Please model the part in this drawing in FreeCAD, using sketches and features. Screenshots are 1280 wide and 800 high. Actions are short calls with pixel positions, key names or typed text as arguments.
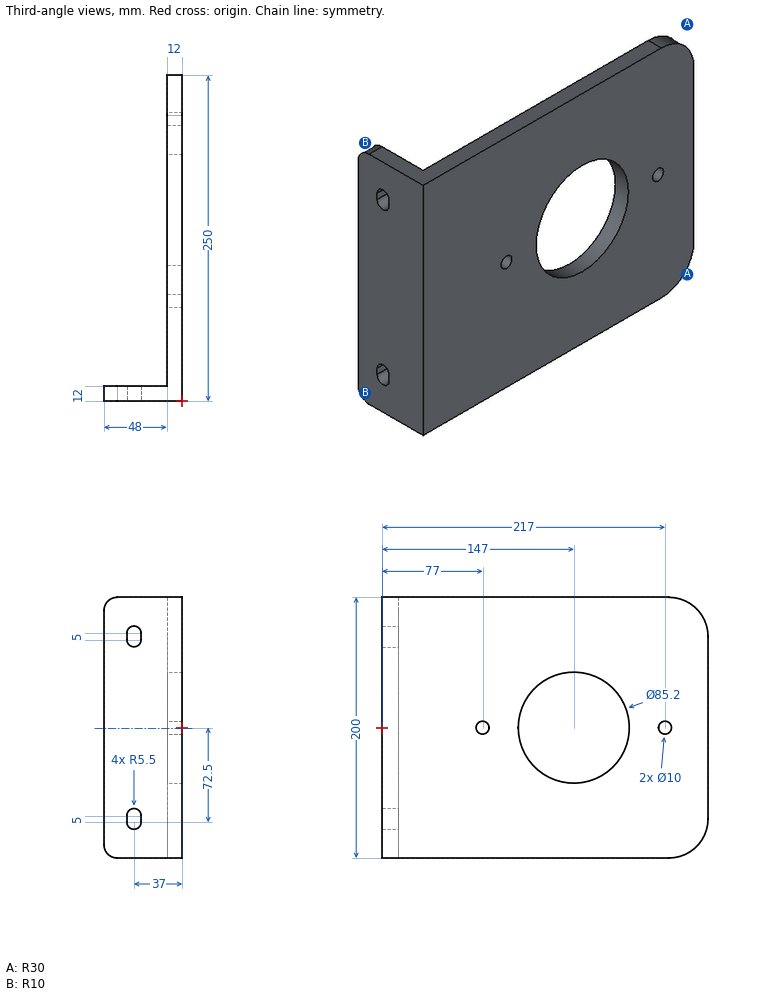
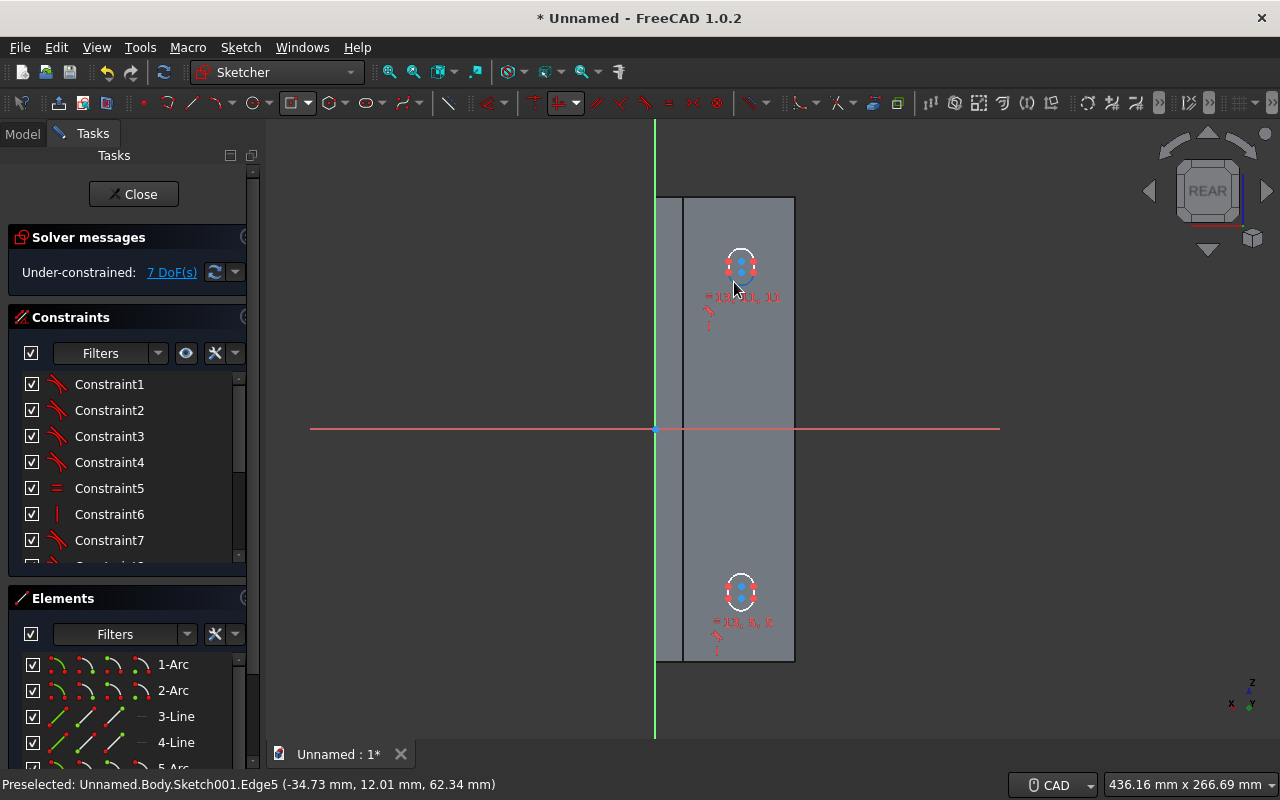
click(741, 587)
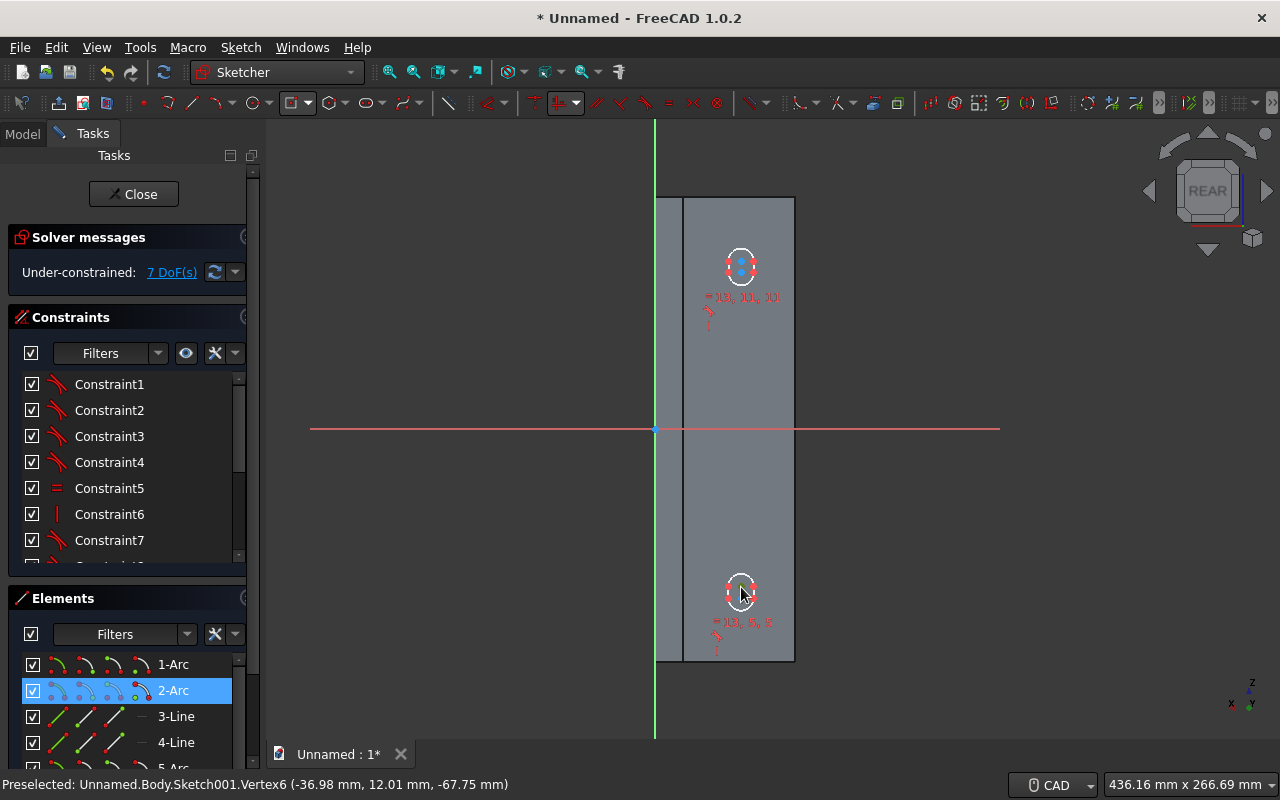
click(741, 273)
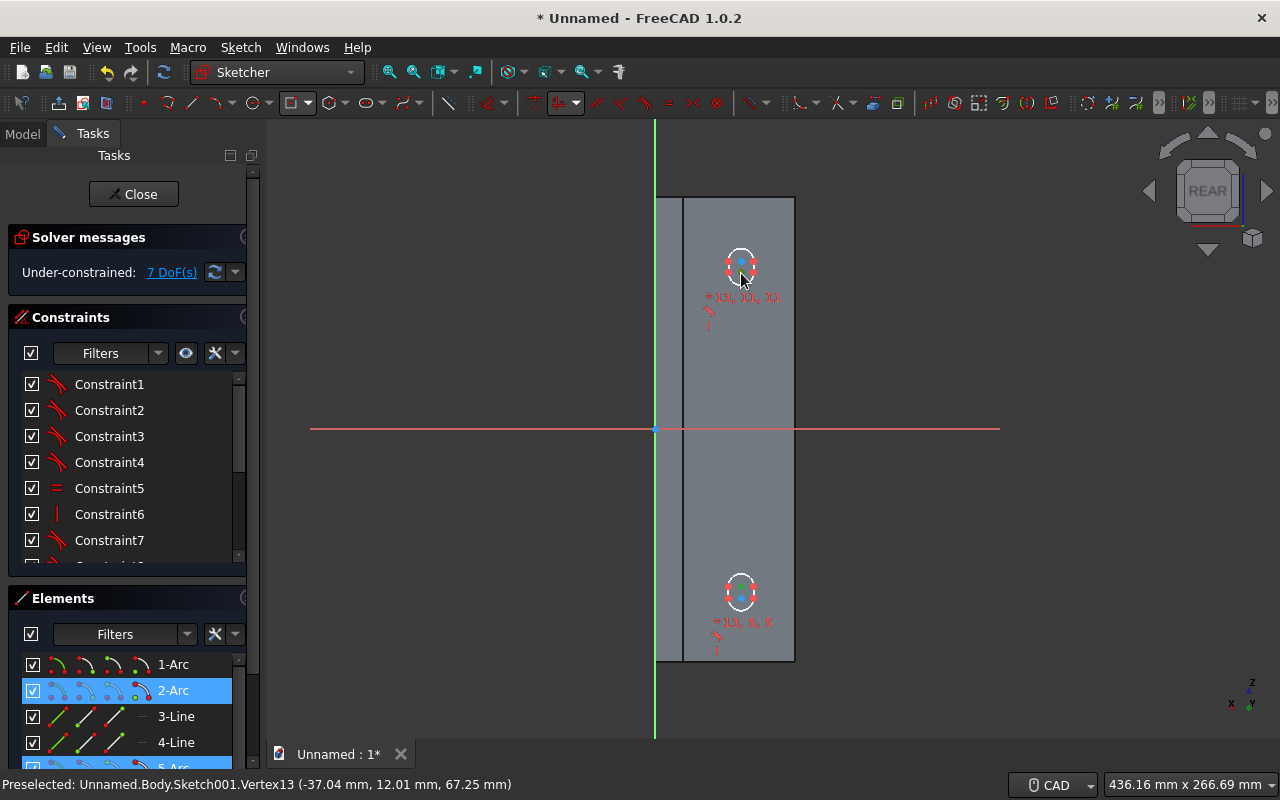
click(353, 429)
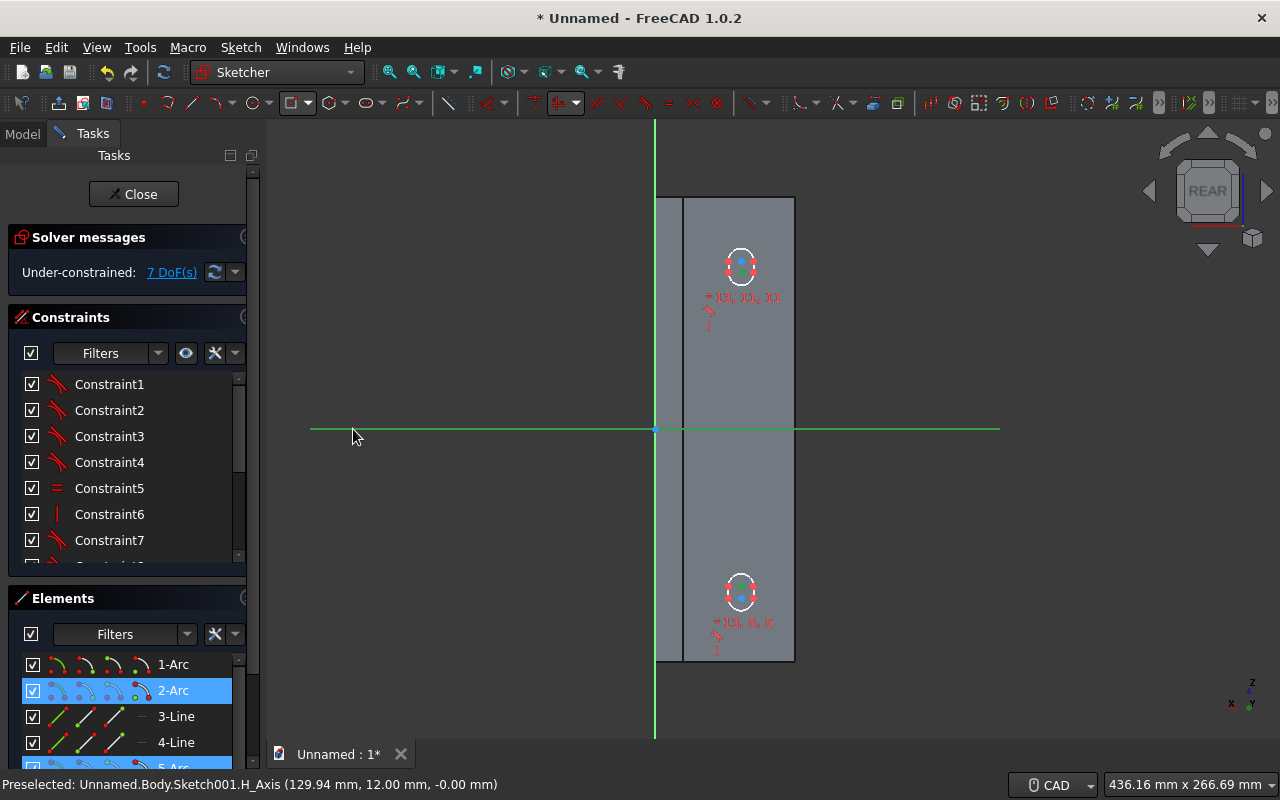
key(s)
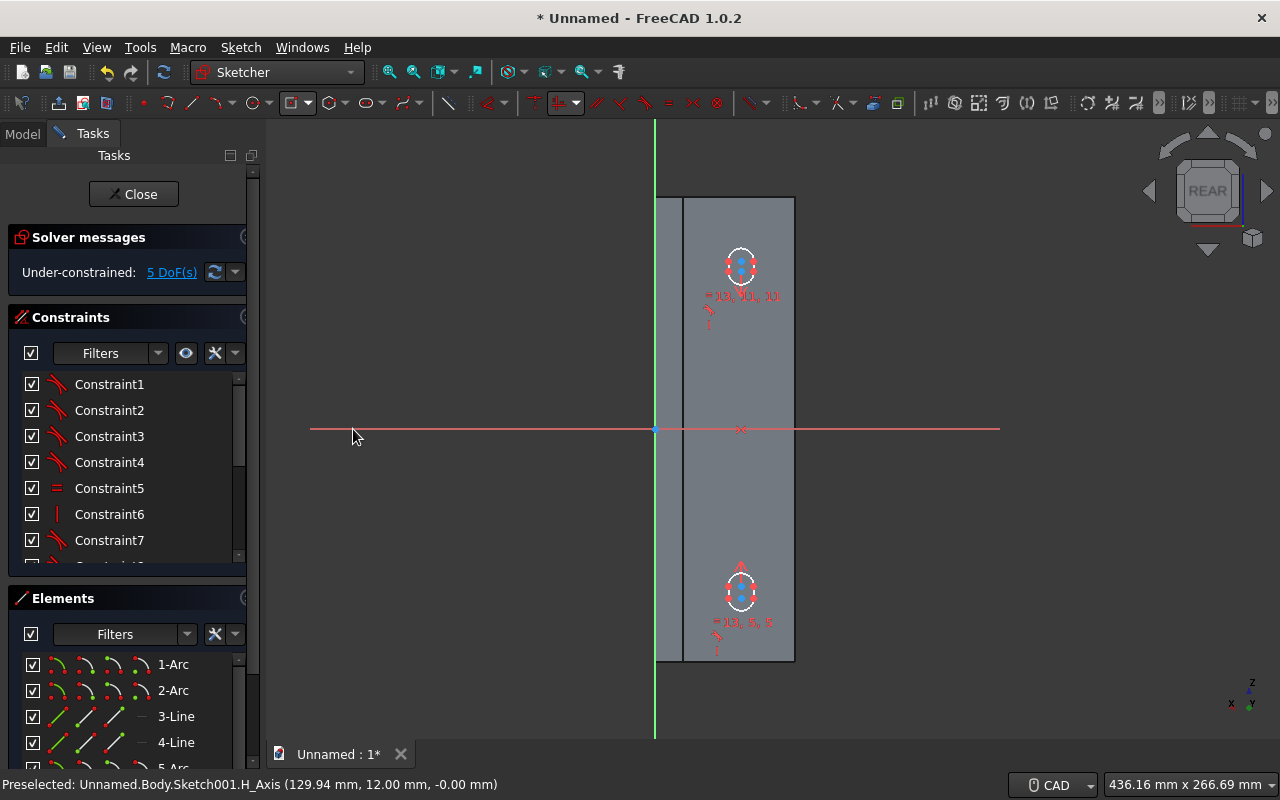
key(d)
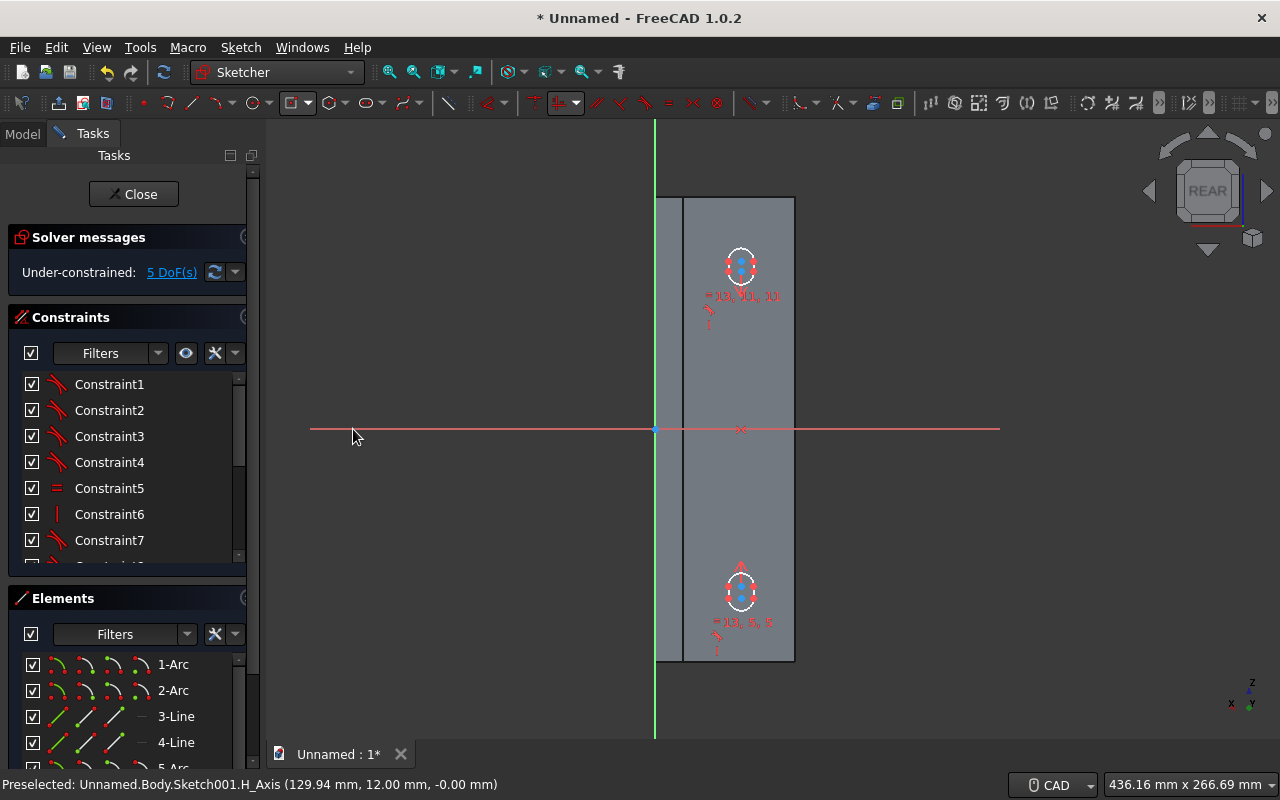
scroll(734, 608, up, 6)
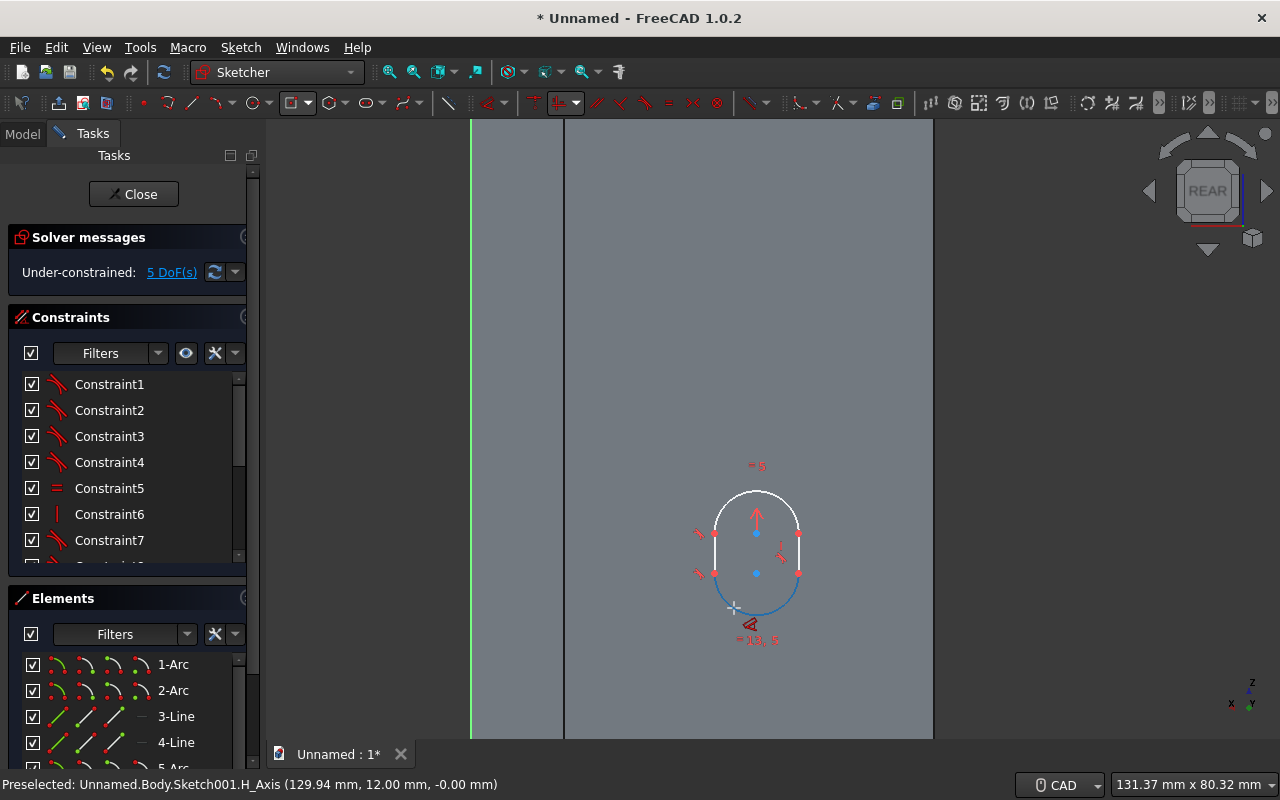
click(732, 607)
click(713, 633)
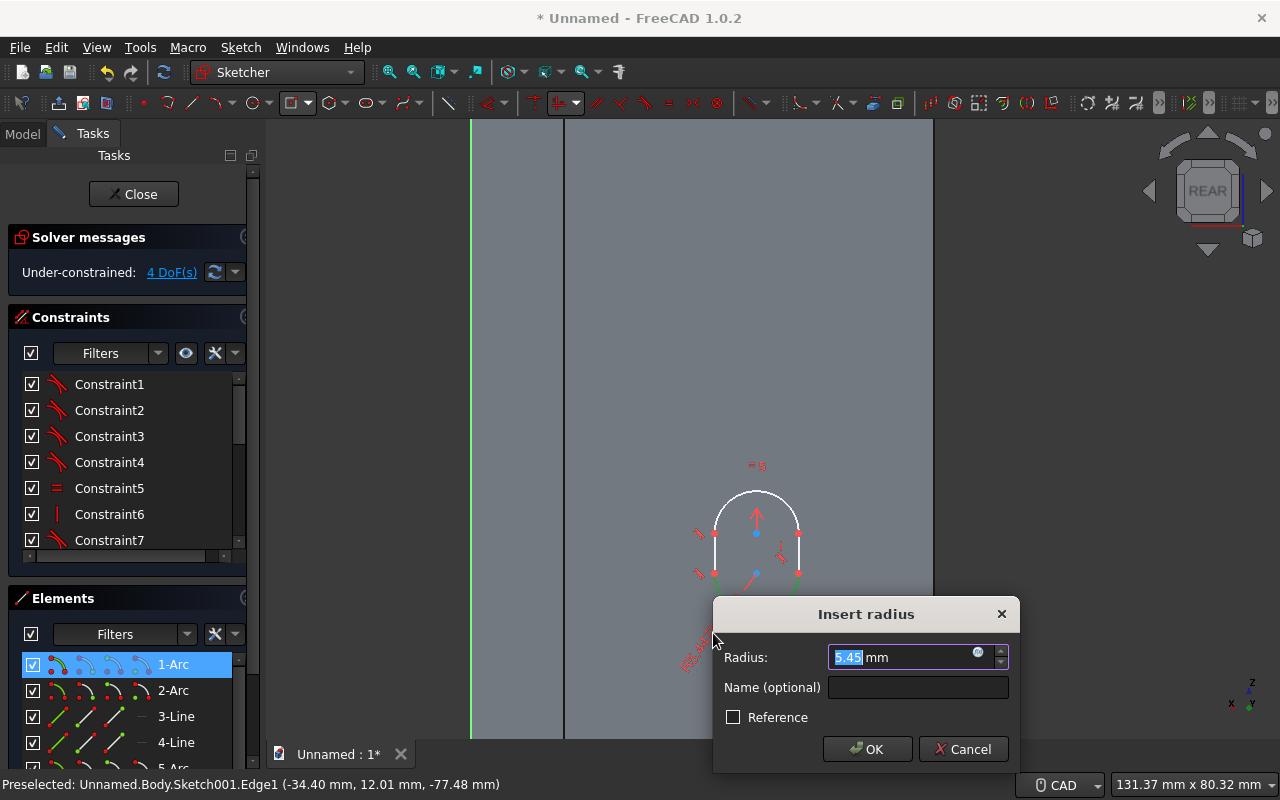
text(5.5)
key(Return)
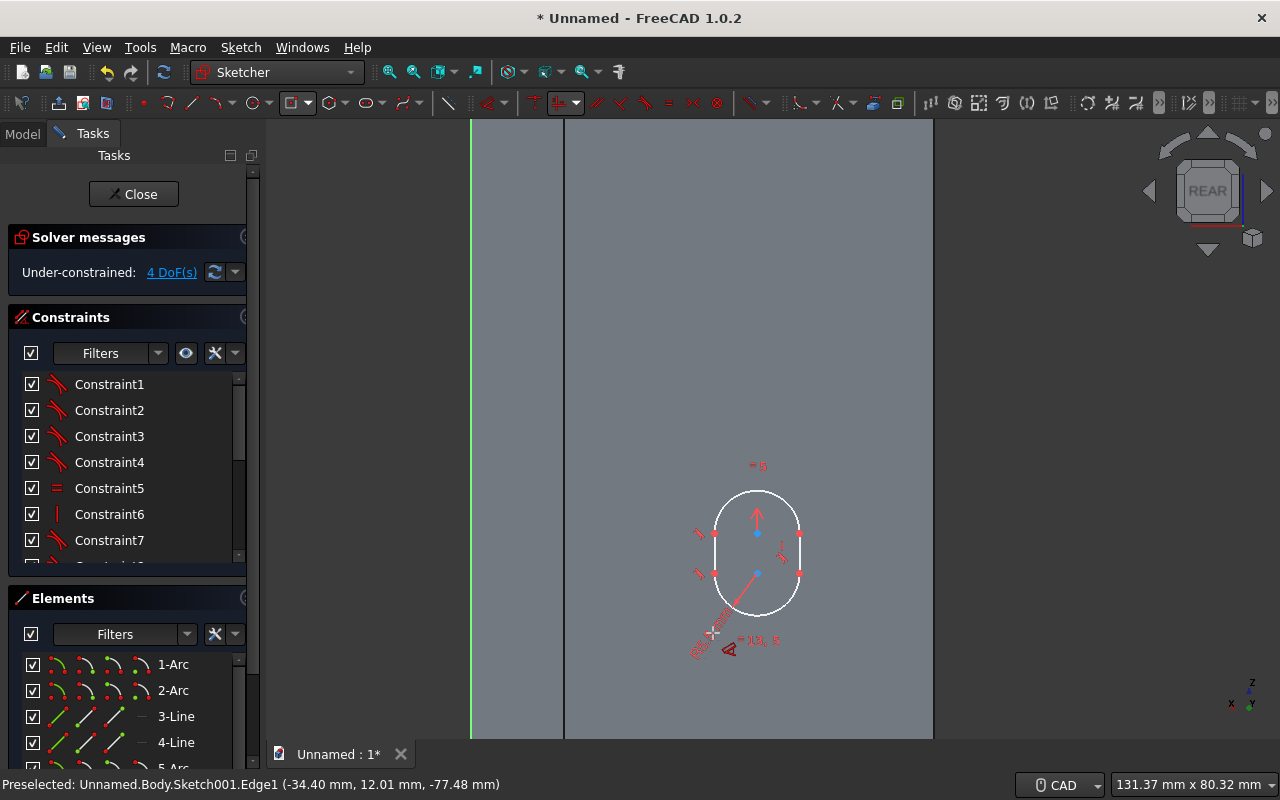
click(715, 561)
click(749, 553)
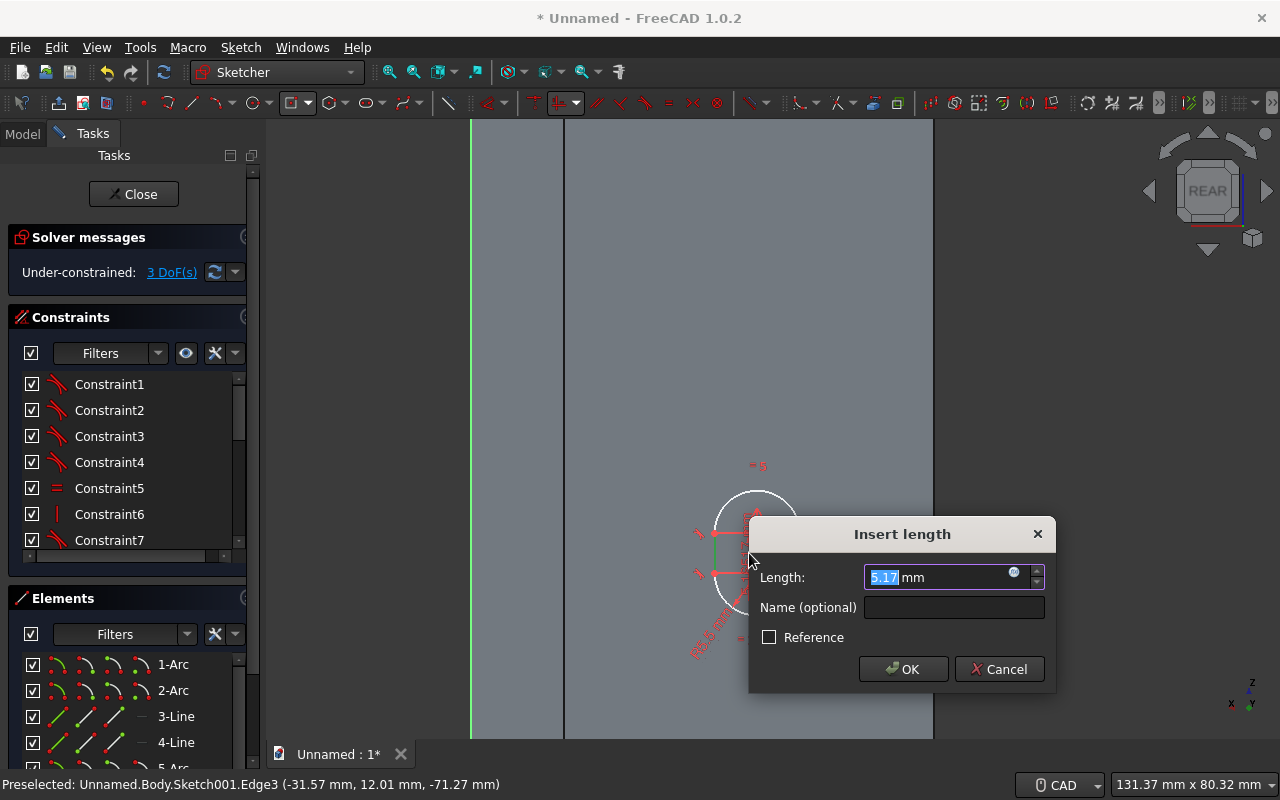
text(5)
key(Return)